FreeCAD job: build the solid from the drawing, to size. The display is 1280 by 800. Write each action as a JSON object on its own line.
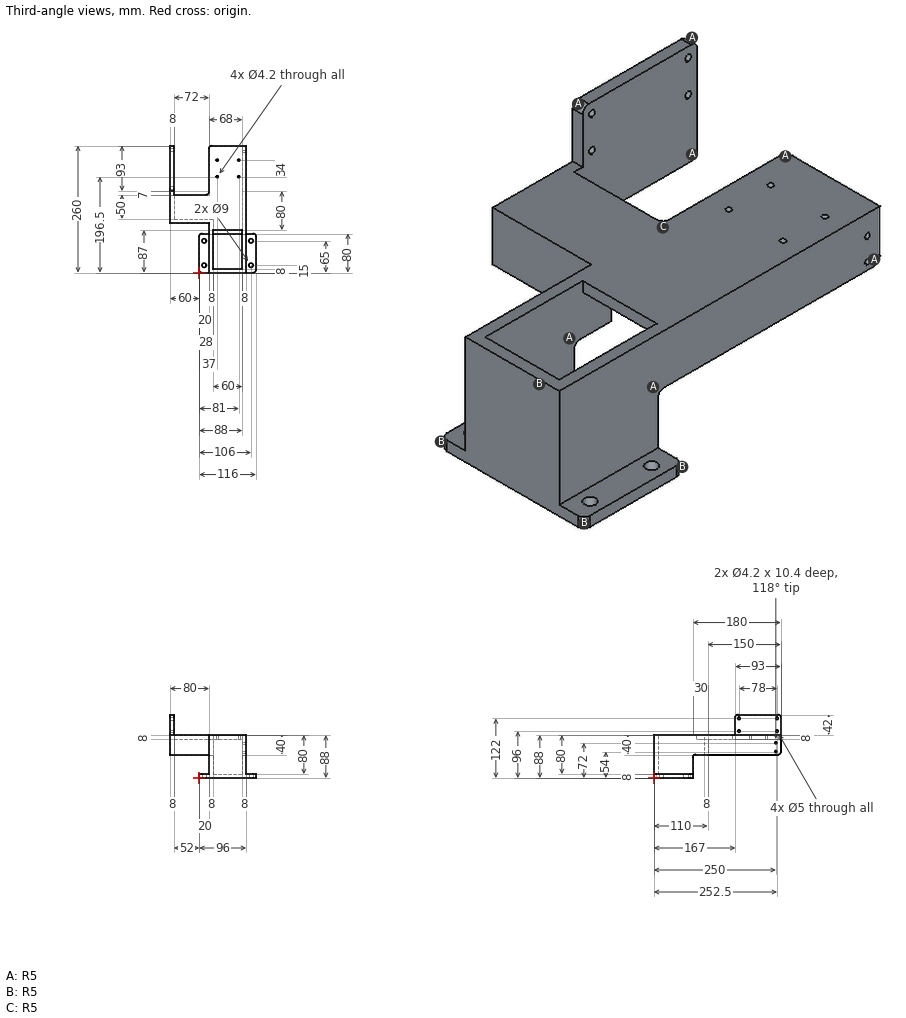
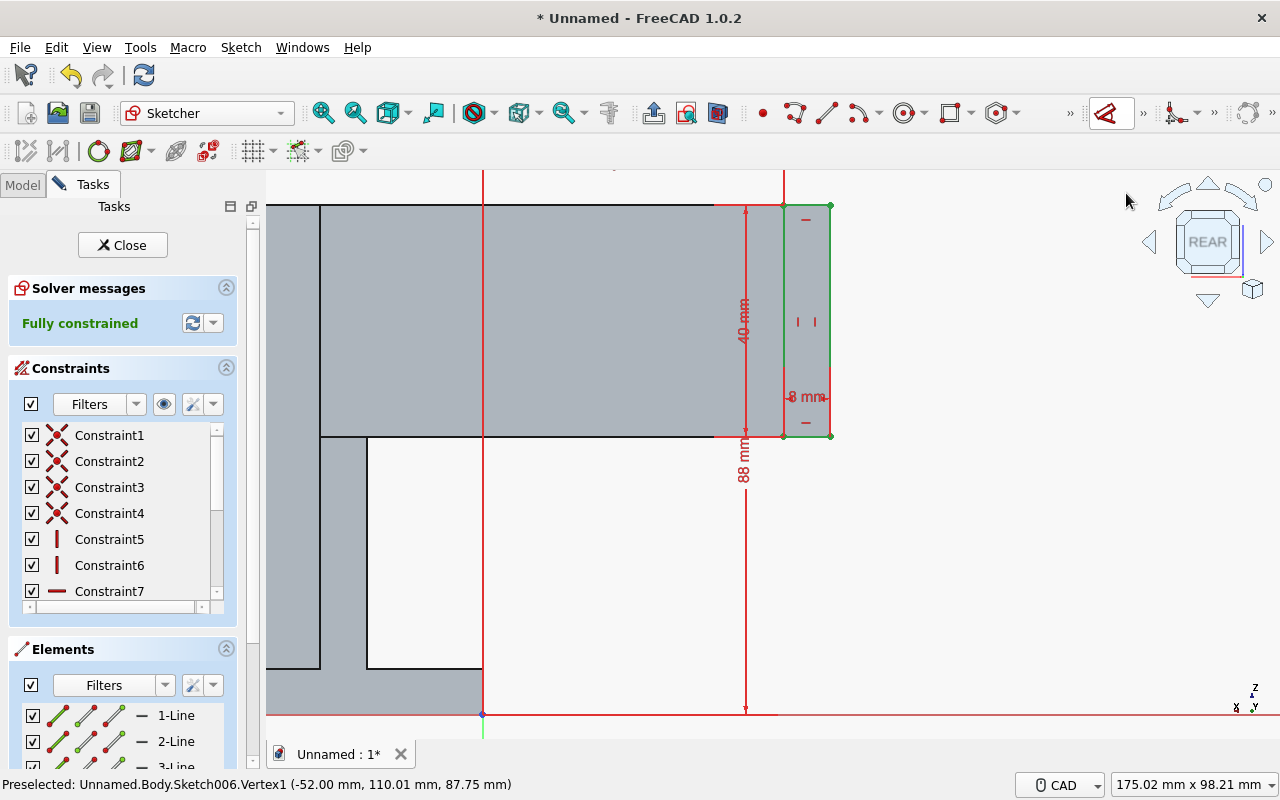
{"action": "left_click", "coordinate": [123, 245]}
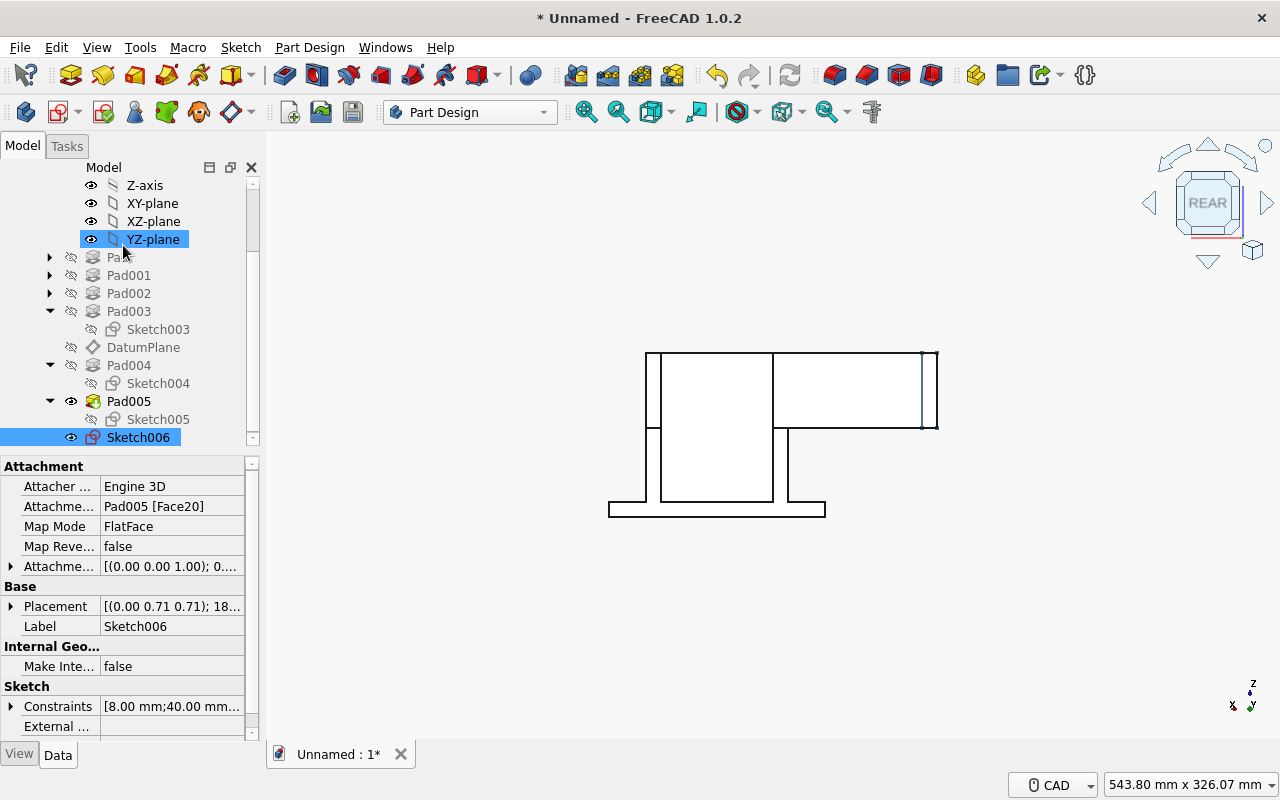
{"action": "left_click", "coordinate": [72, 76]}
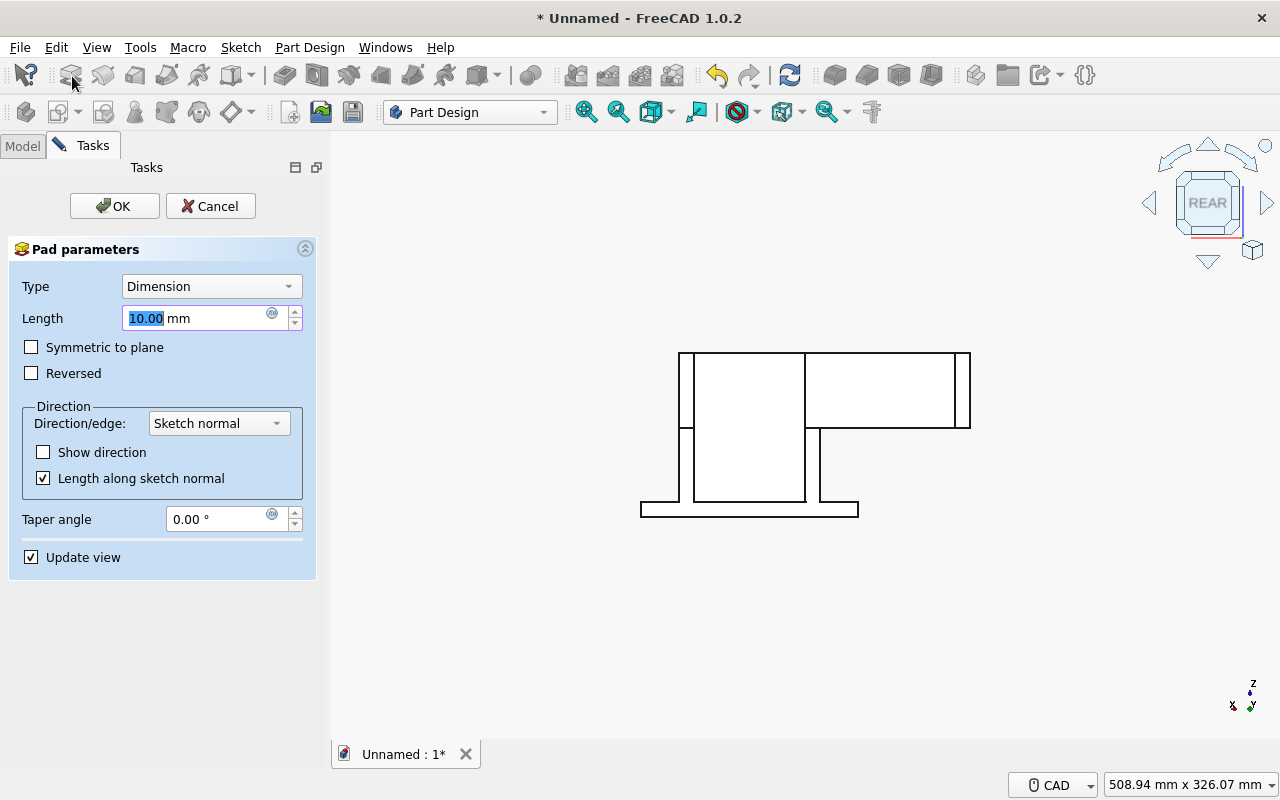
{"action": "type", "text": "150"}
{"action": "key", "text": "Tab"}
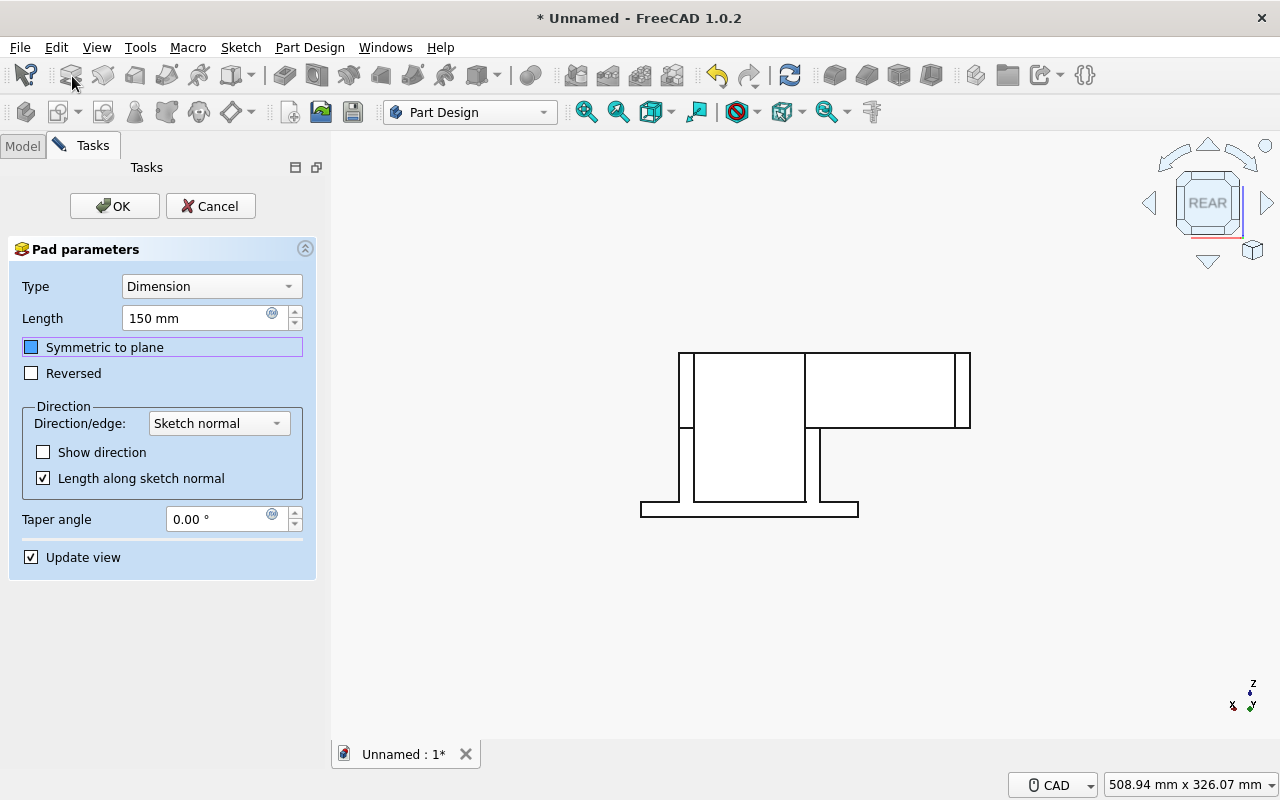
{"action": "left_click", "coordinate": [115, 206]}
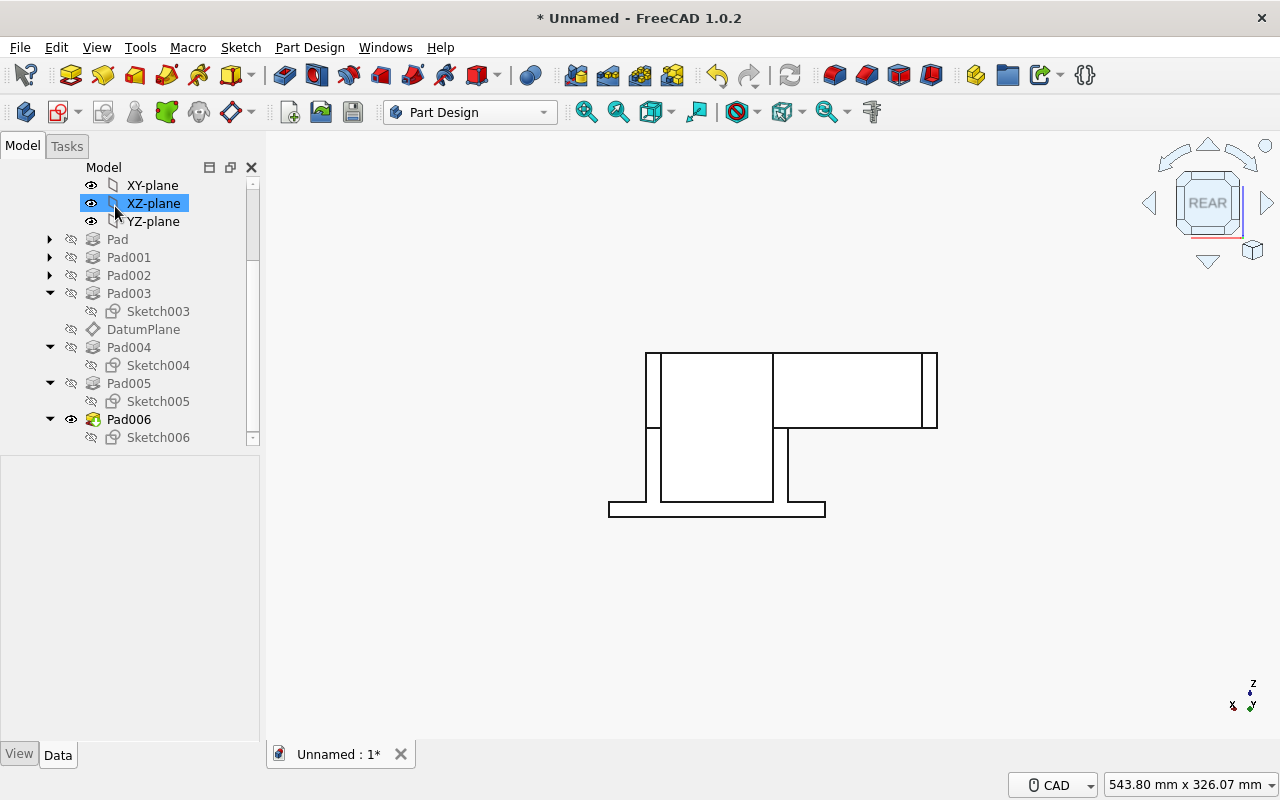
{"action": "left_click", "coordinate": [588, 112]}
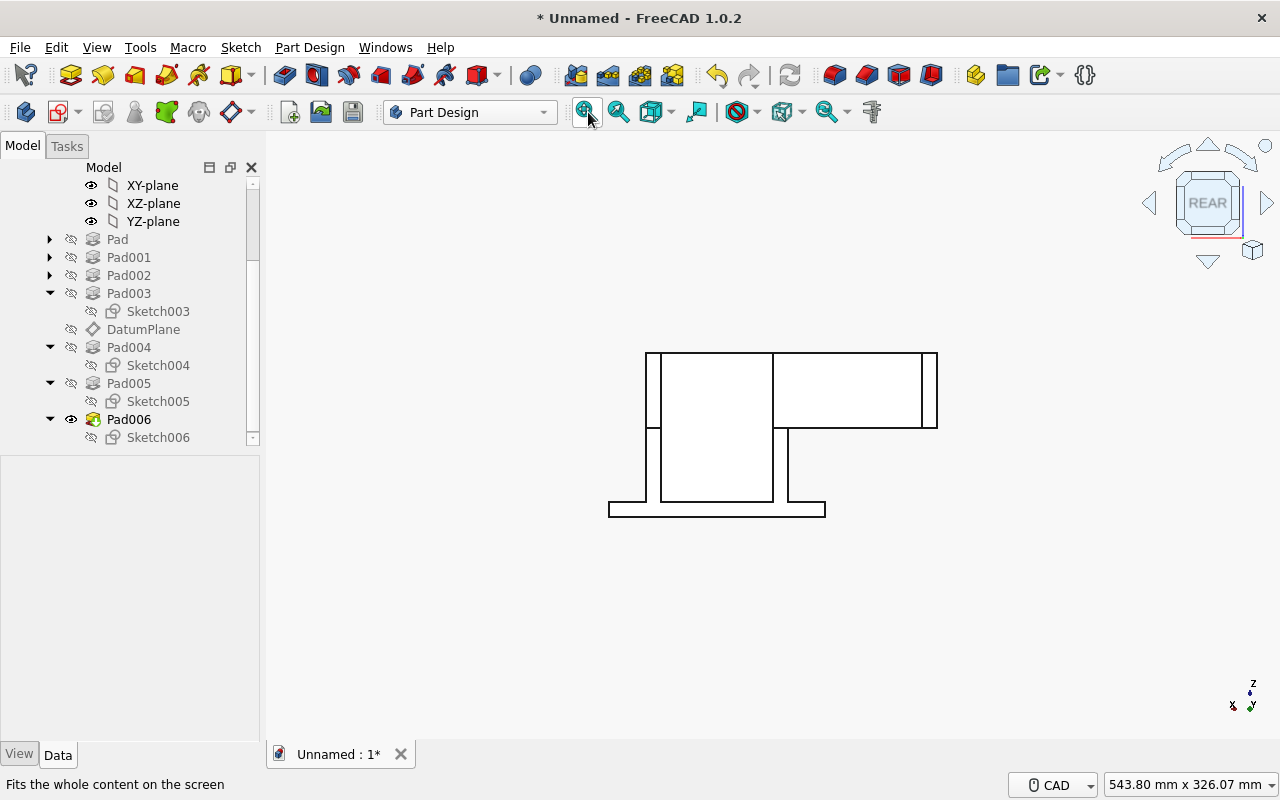
{"action": "scroll", "coordinate": [160, 307], "scroll_direction": "down", "scroll_amount": 3}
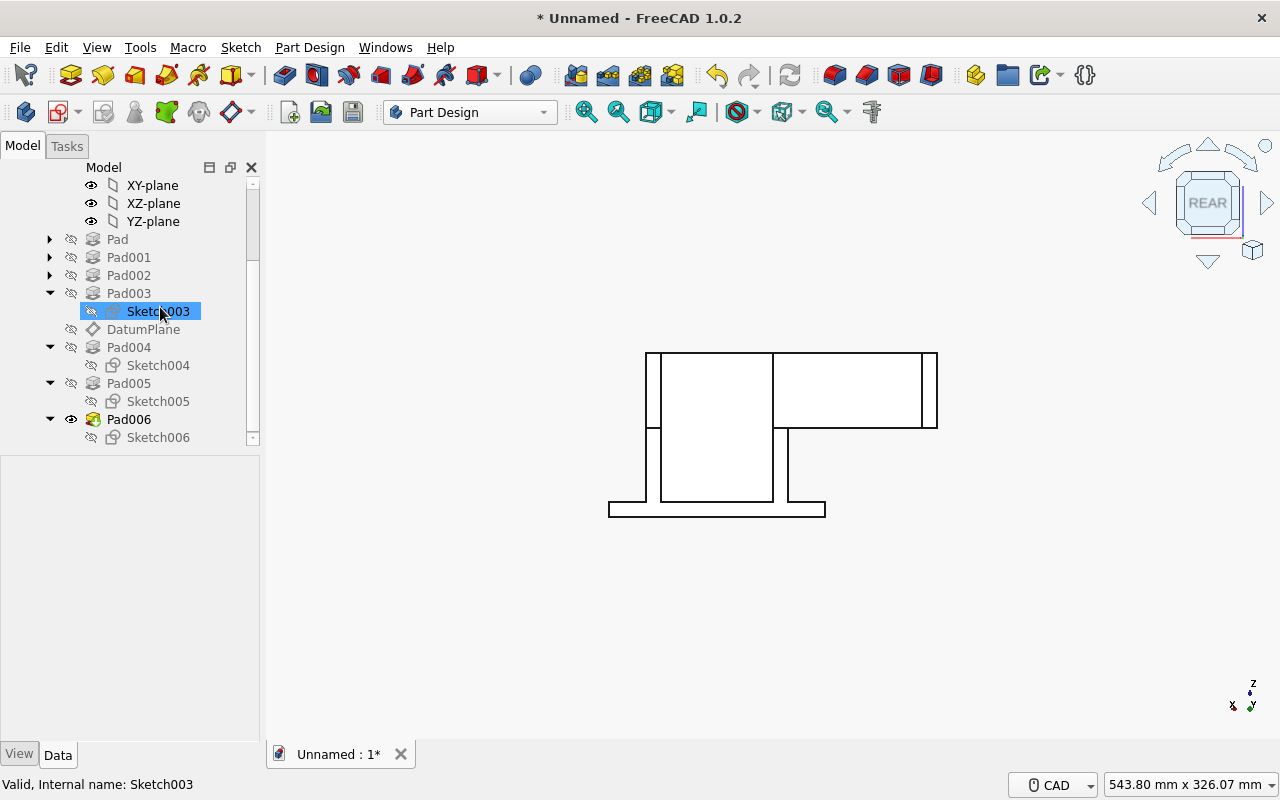
{"action": "scroll", "coordinate": [160, 307], "scroll_direction": "up", "scroll_amount": 15}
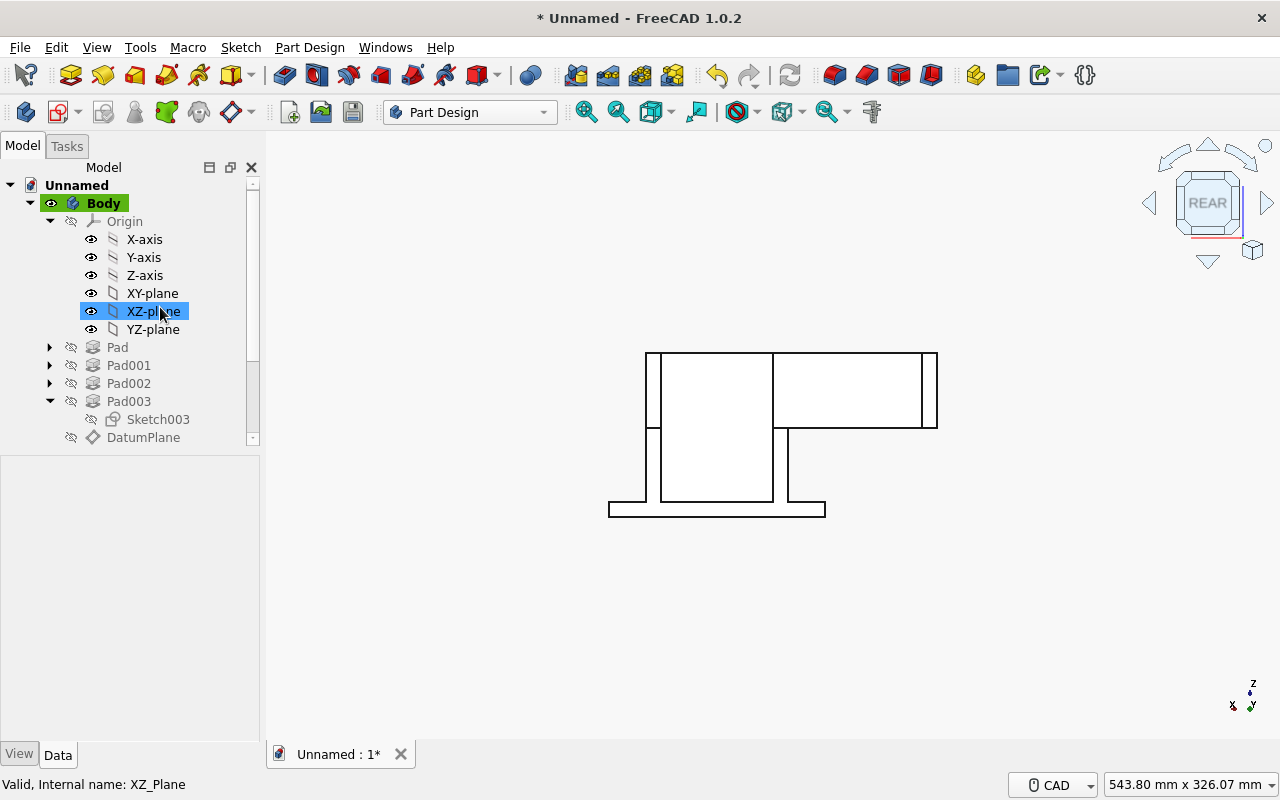
{"action": "left_click", "coordinate": [136, 329]}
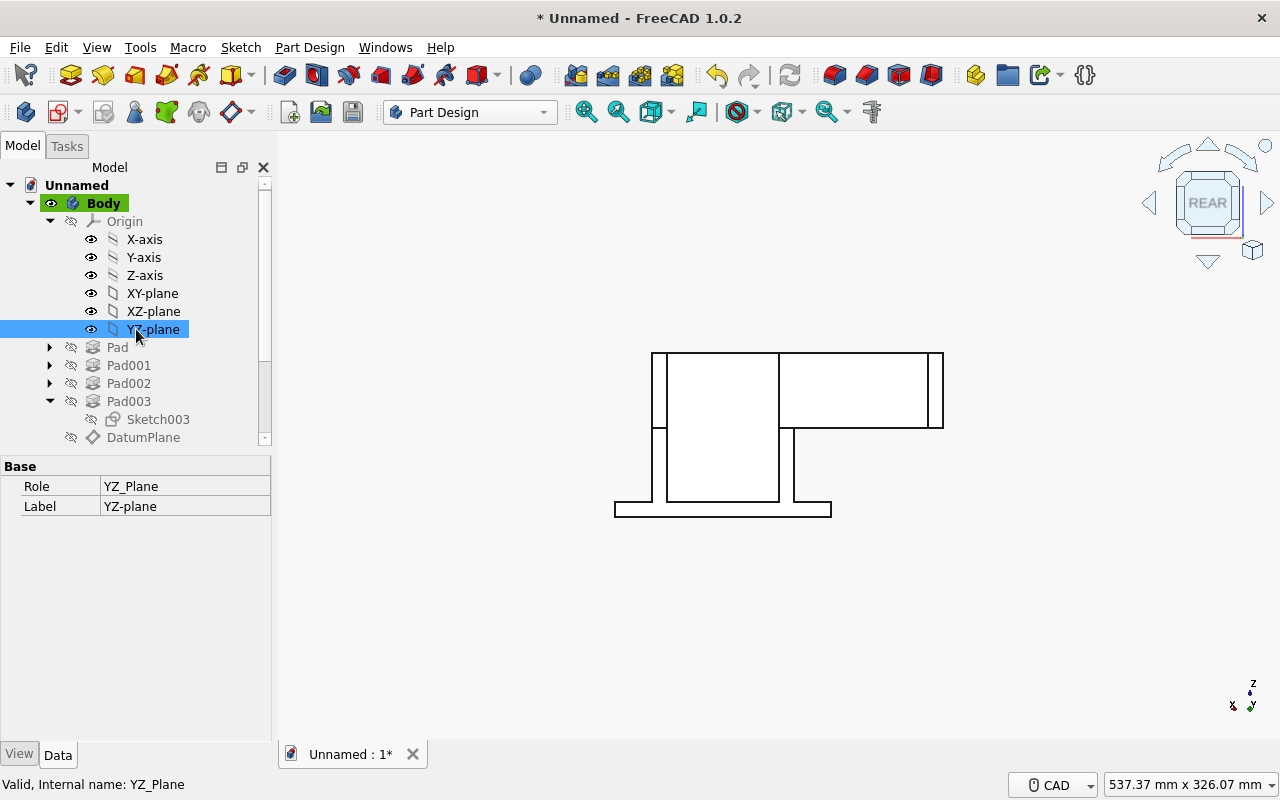
{"action": "left_click", "coordinate": [232, 112]}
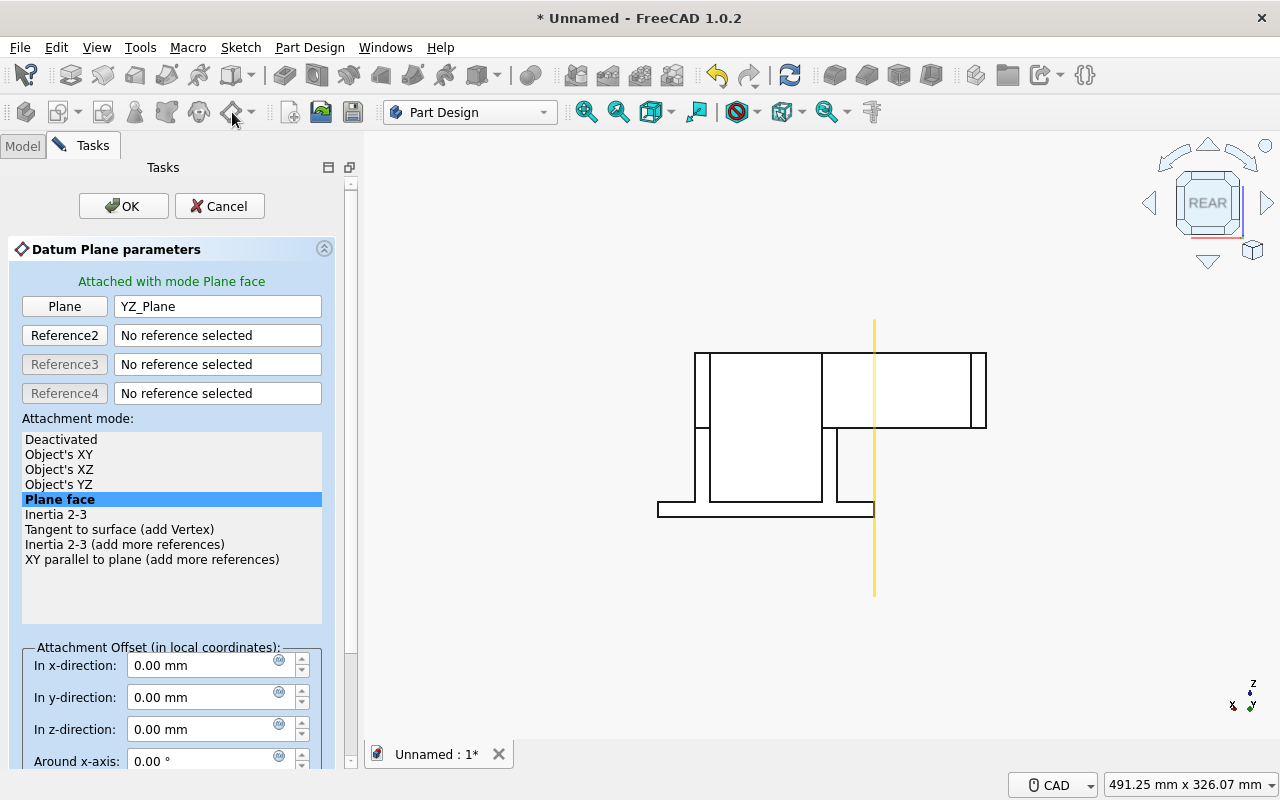
{"action": "triple_click", "coordinate": [210, 729]}